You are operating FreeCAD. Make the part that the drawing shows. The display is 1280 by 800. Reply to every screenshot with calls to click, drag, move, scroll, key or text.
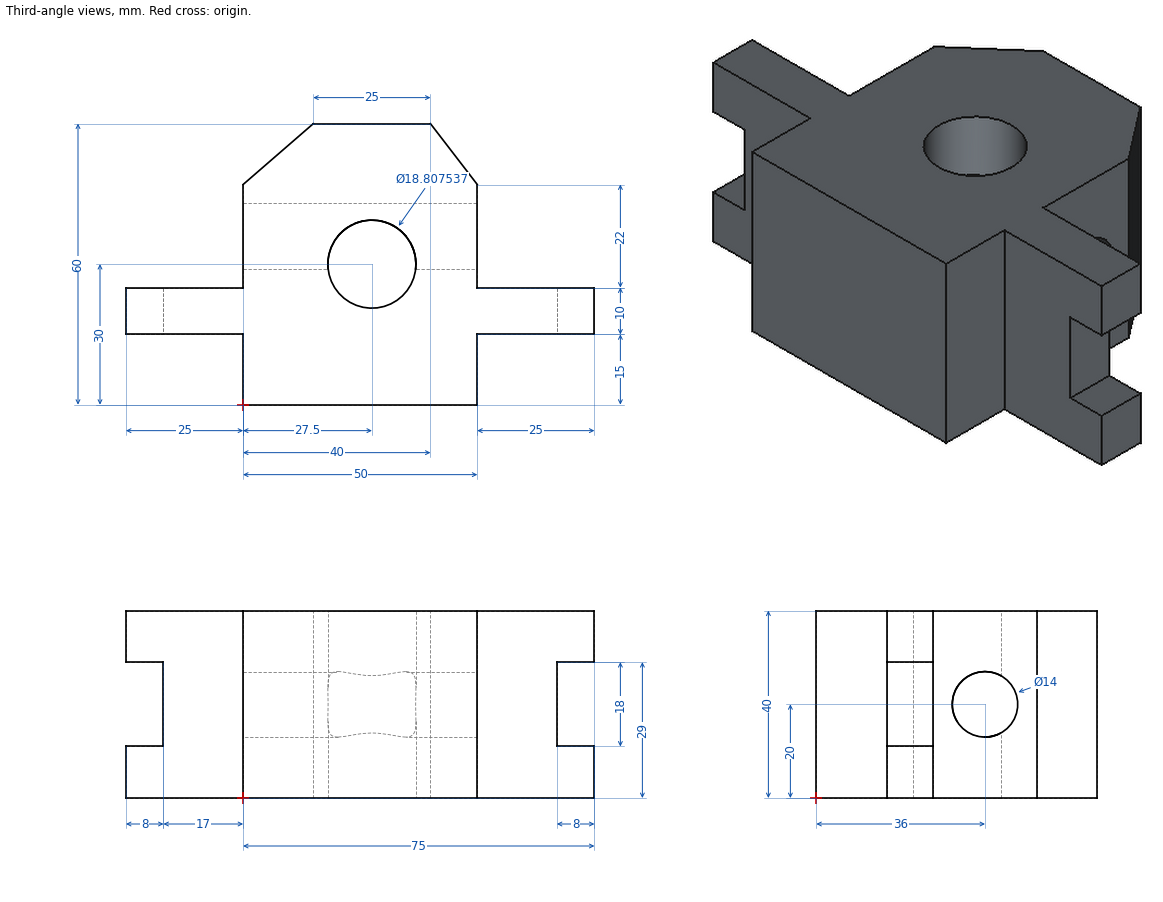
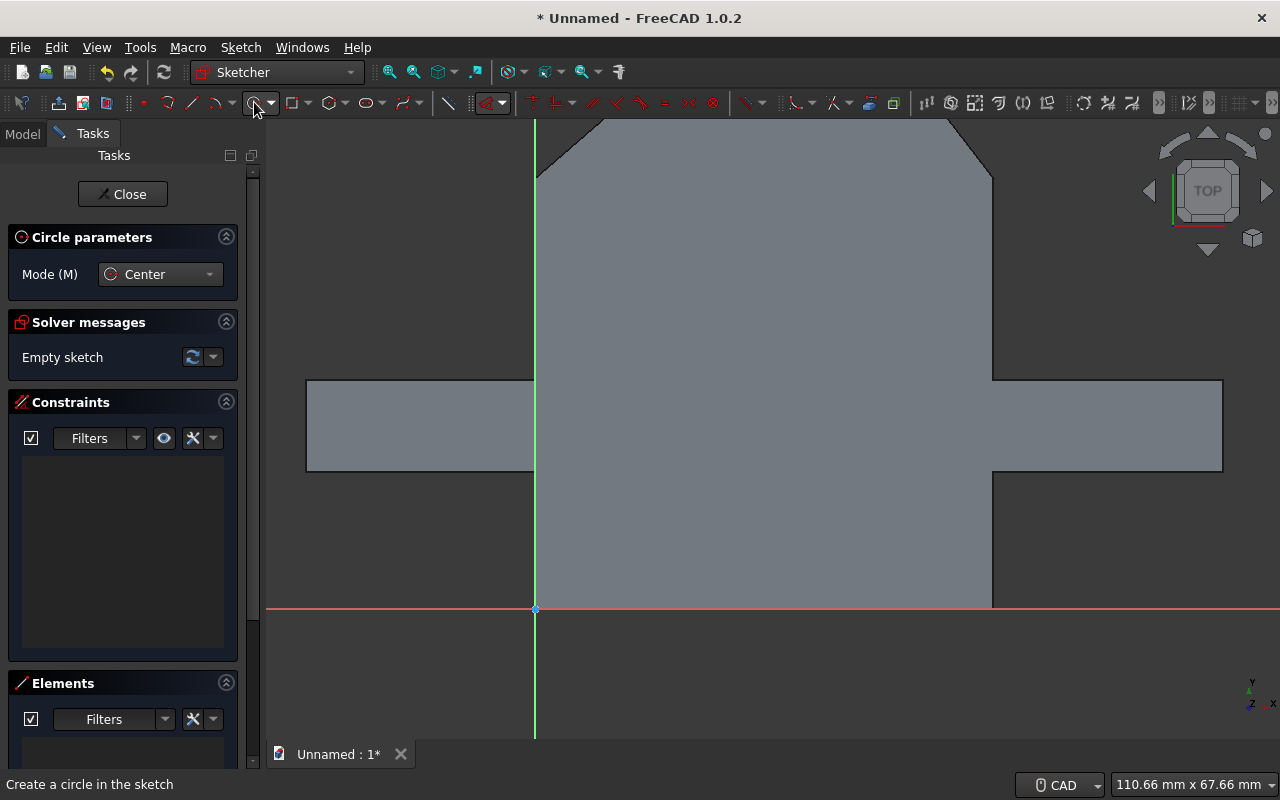
click(787, 334)
move(848, 273)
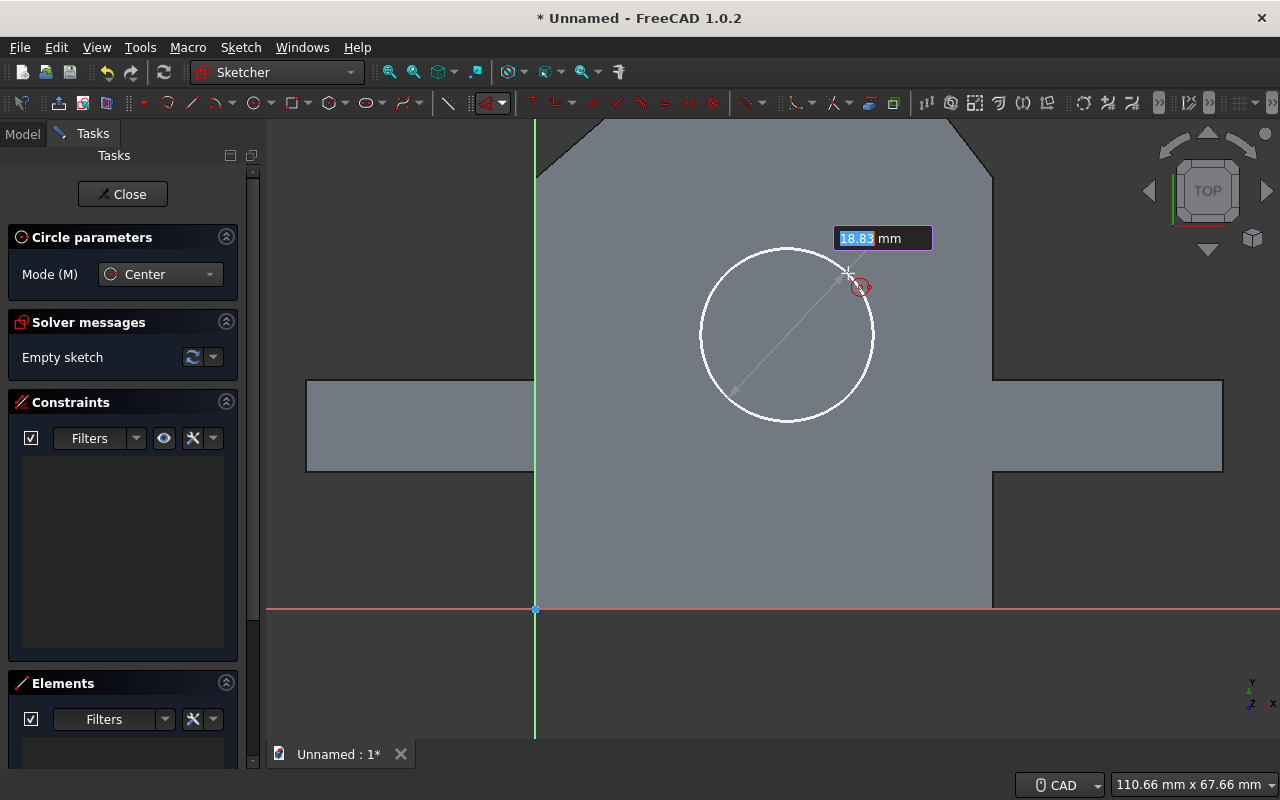
text(18.807537)
key(Return)
key(Escape)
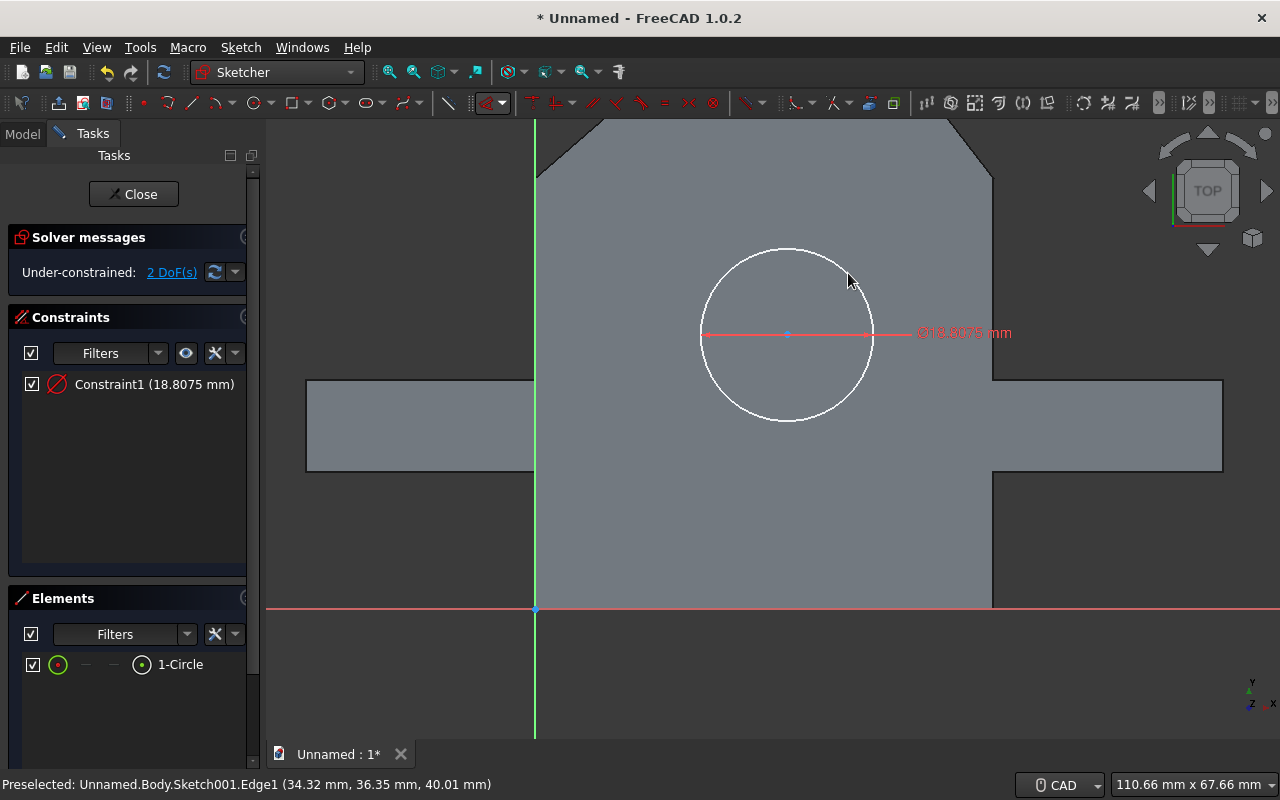
click(787, 335)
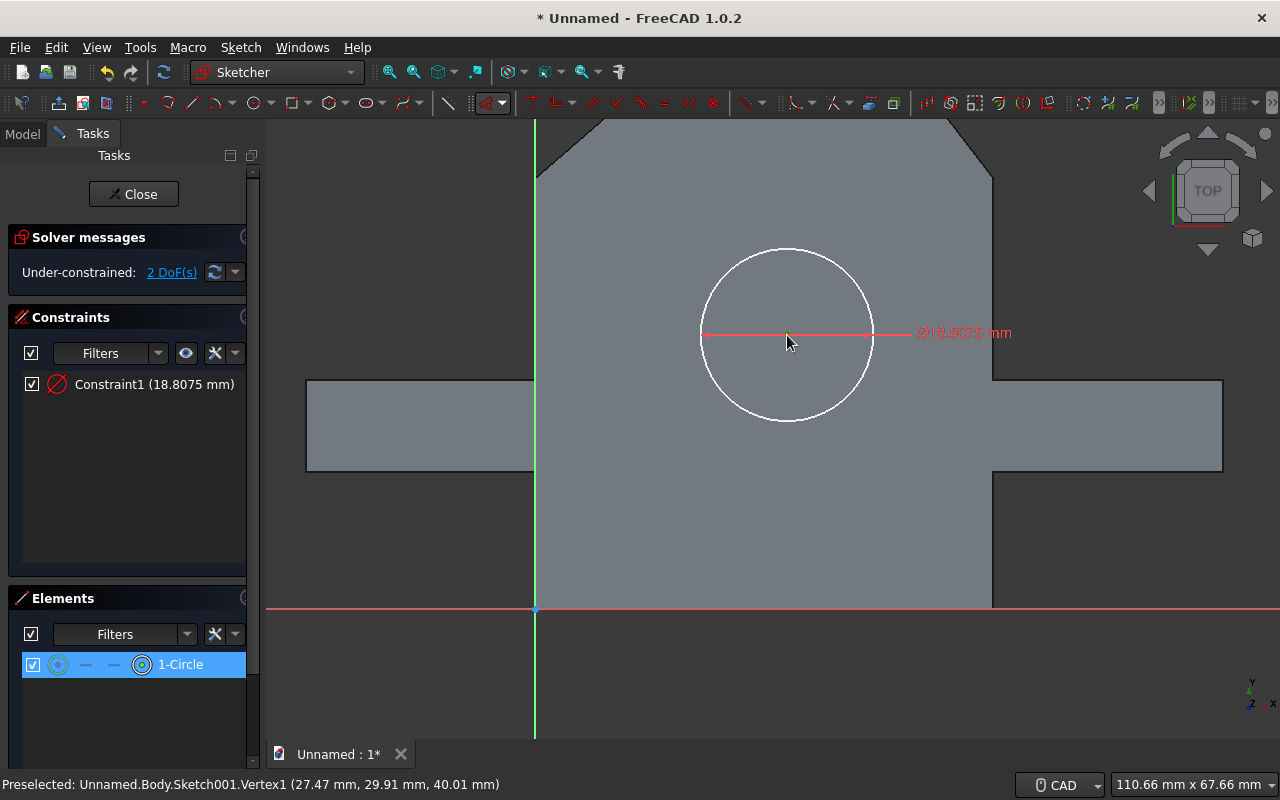
click(504, 104)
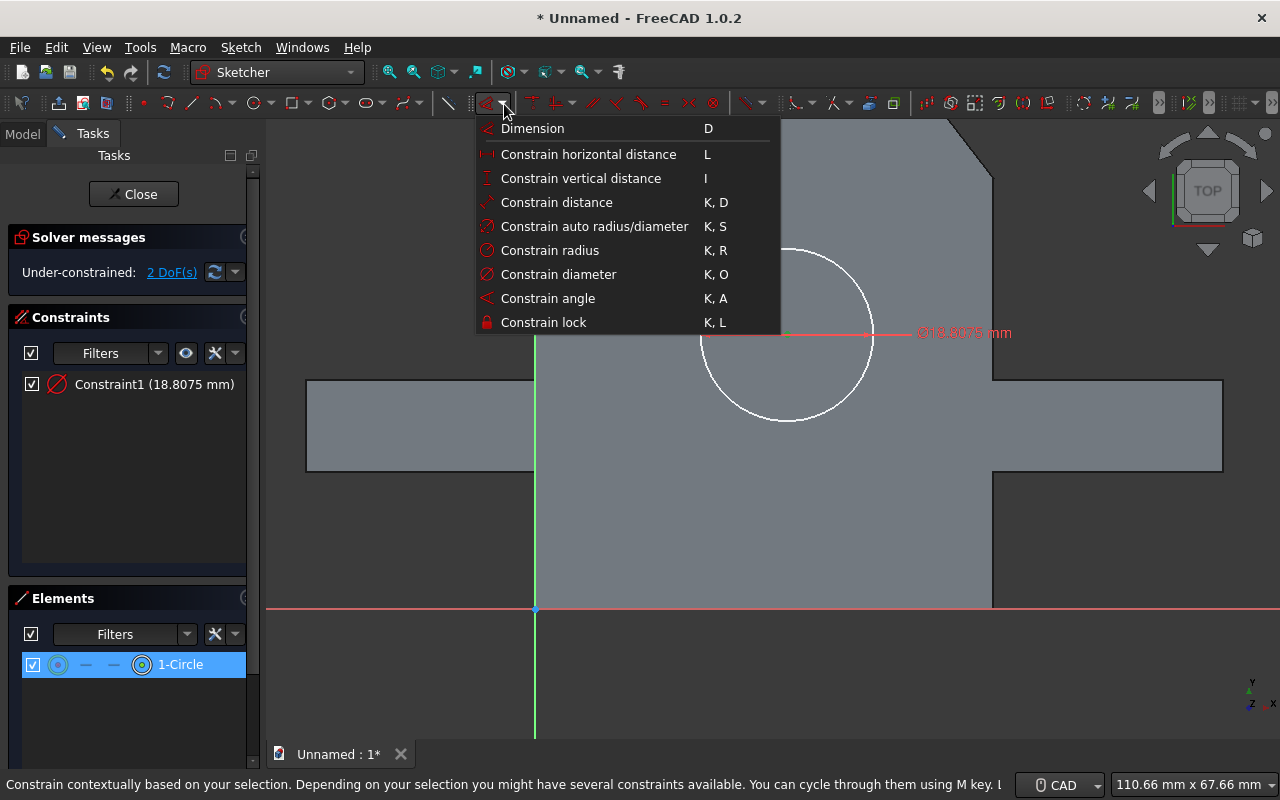
click(628, 178)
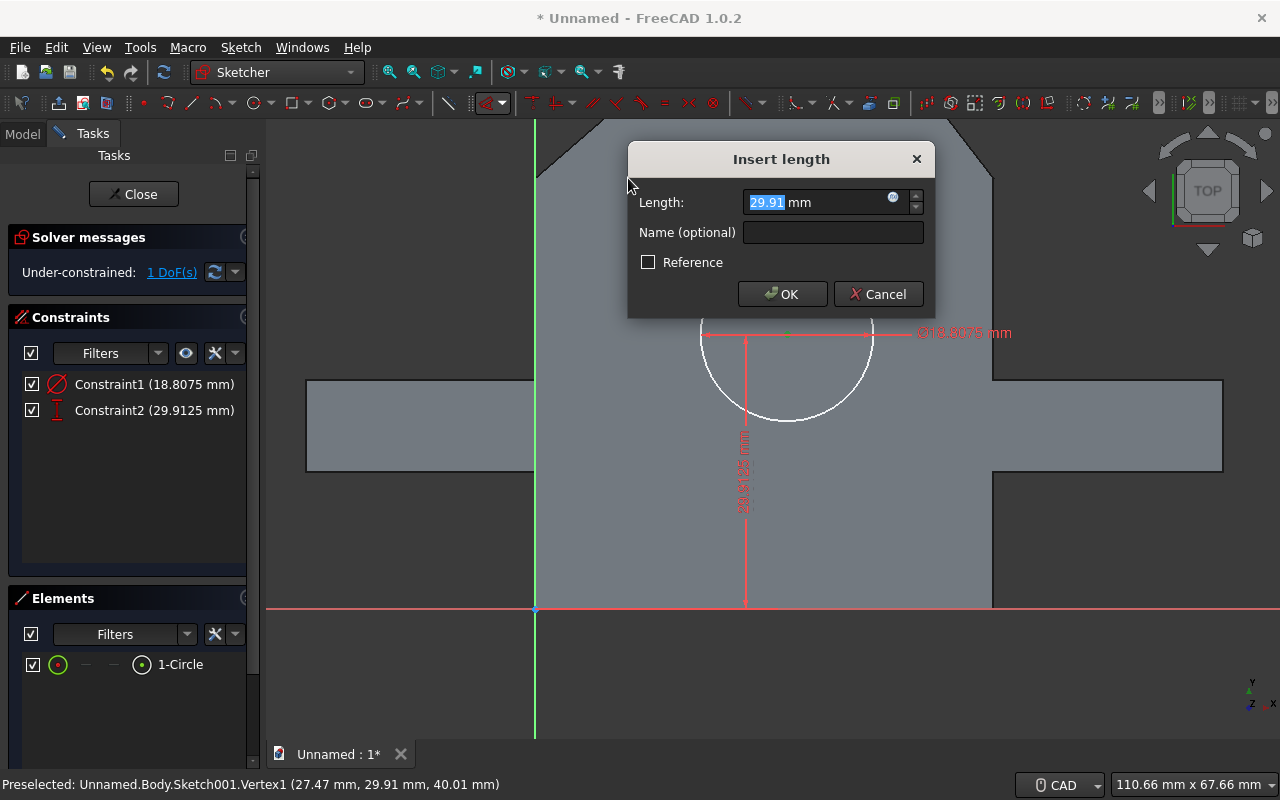
text(30)
key(Return)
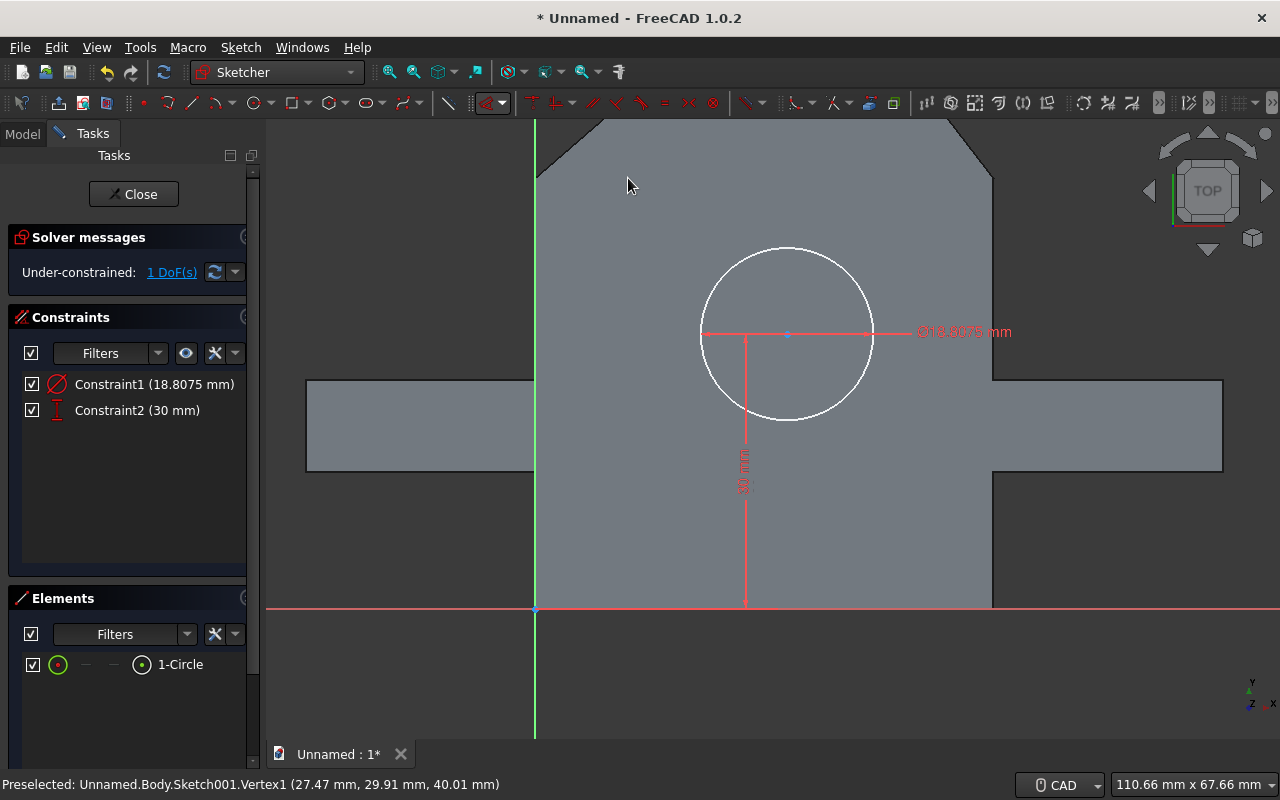
click(787, 334)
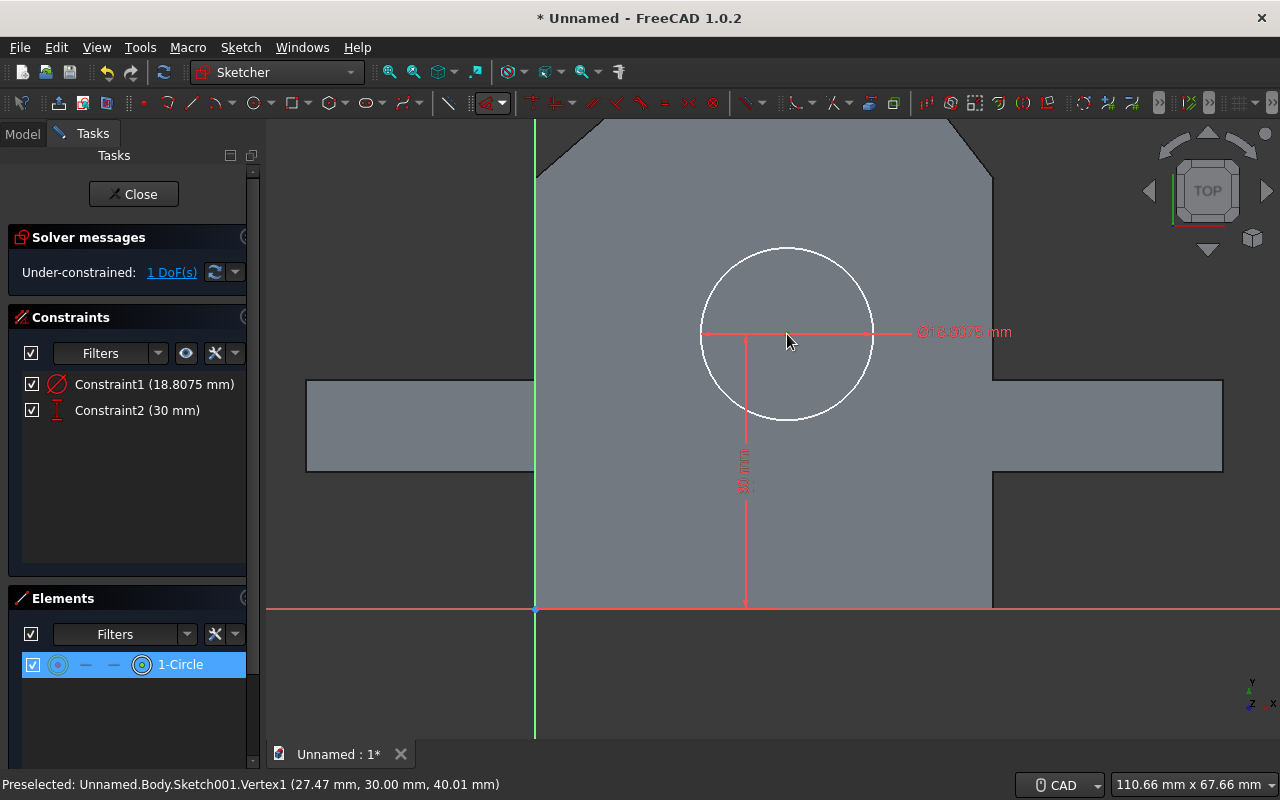
key(l)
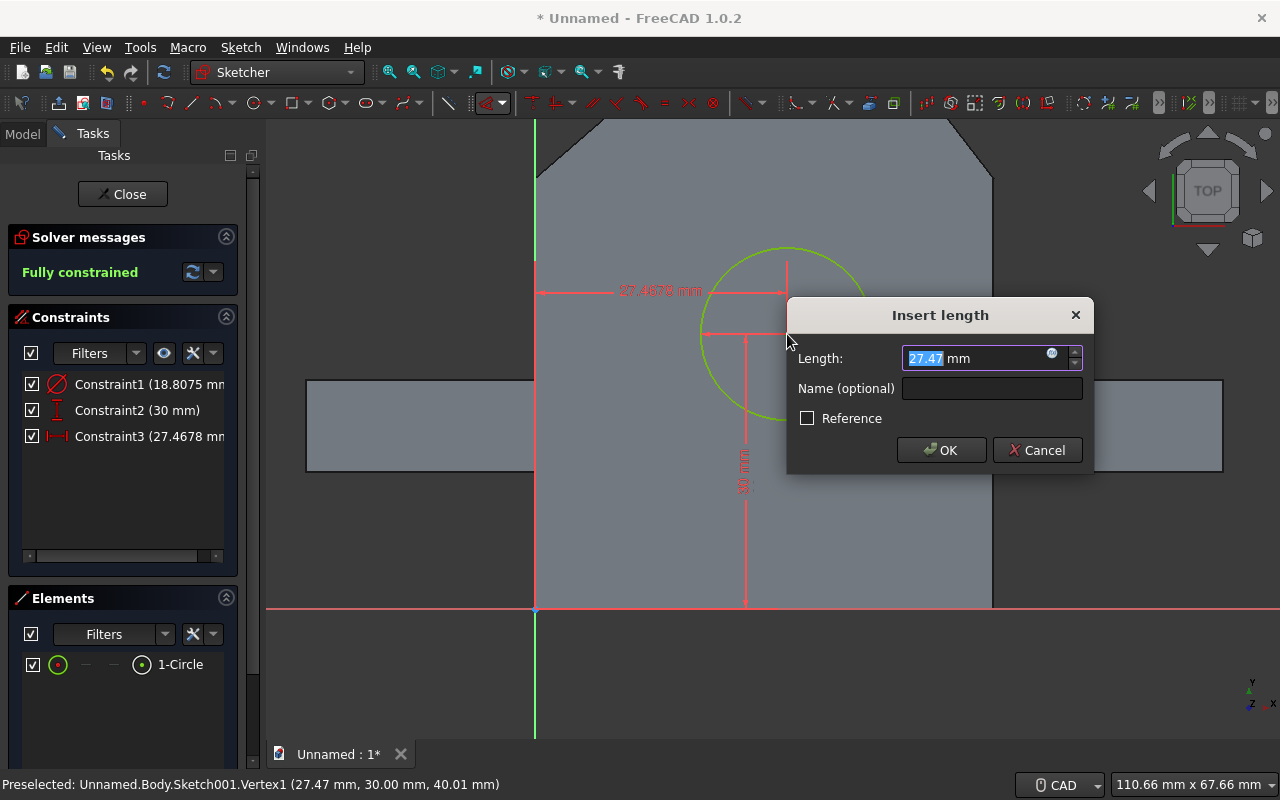
text(27.5)
key(Return)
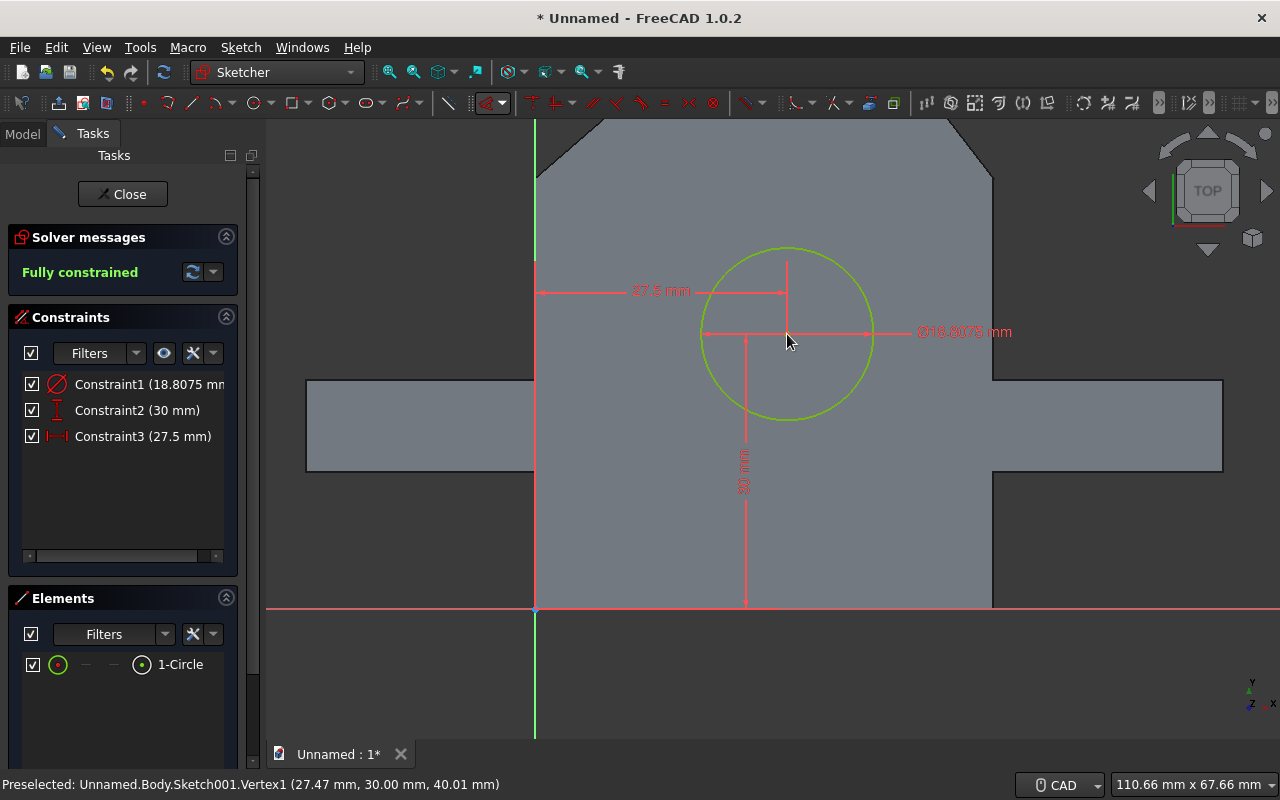
click(123, 194)